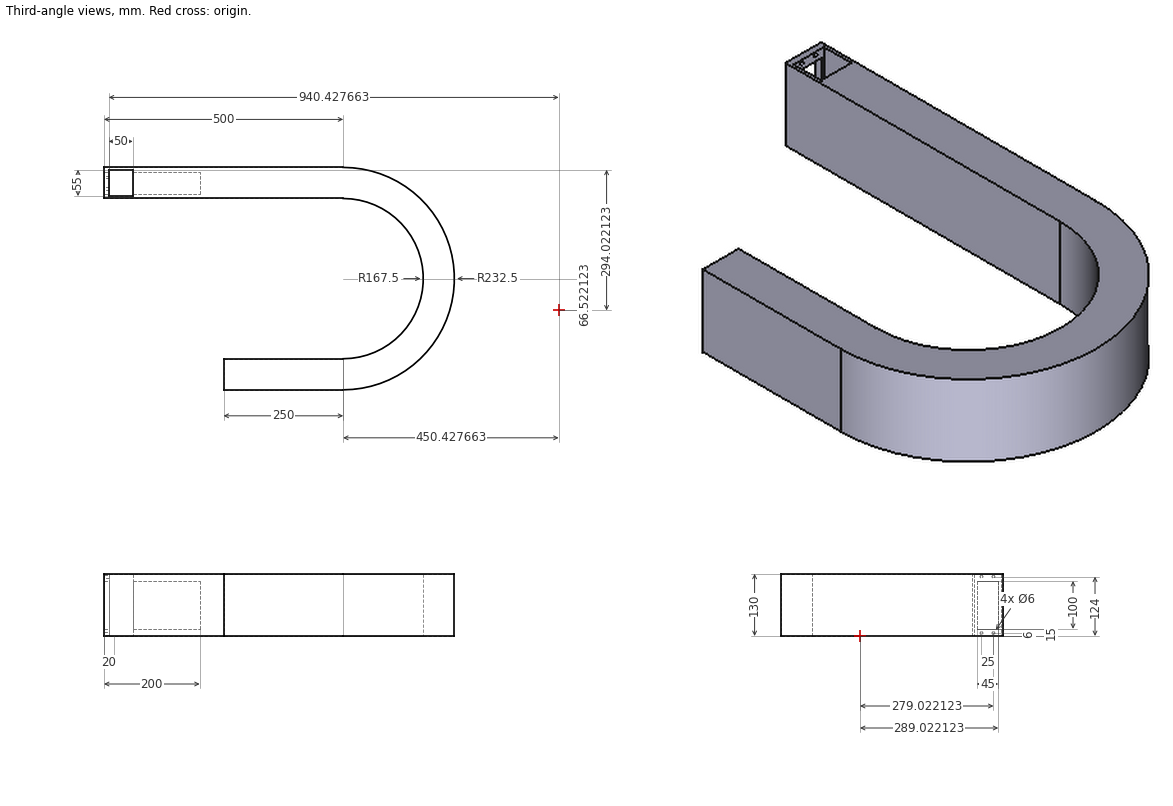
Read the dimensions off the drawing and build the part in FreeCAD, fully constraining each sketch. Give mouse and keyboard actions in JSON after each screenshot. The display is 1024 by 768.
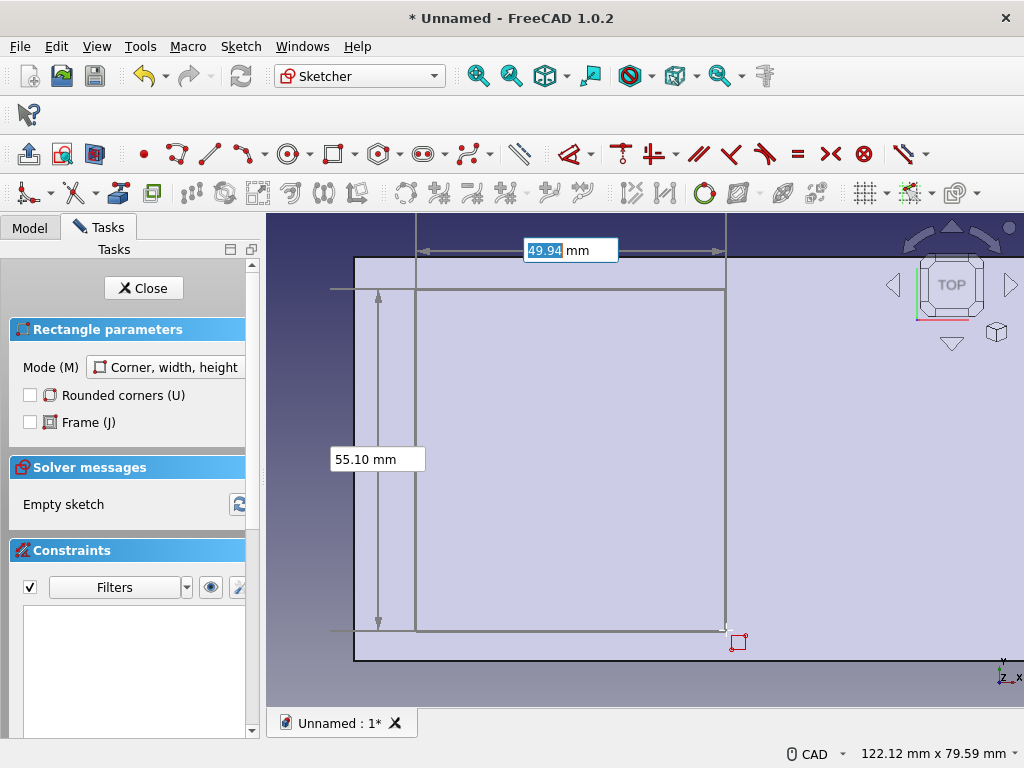
{"action": "type", "text": "50"}
{"action": "key", "text": "Tab"}
{"action": "type", "text": "55"}
{"action": "key", "text": "Return"}
{"action": "key", "text": "Escape"}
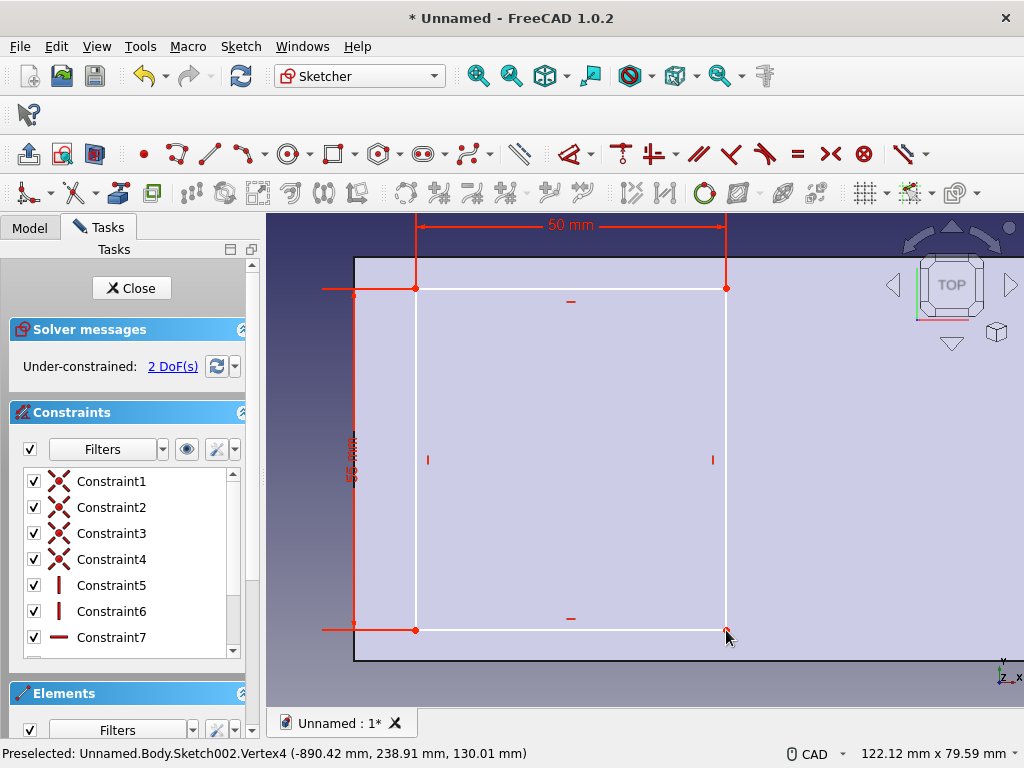
{"action": "key", "text": "d"}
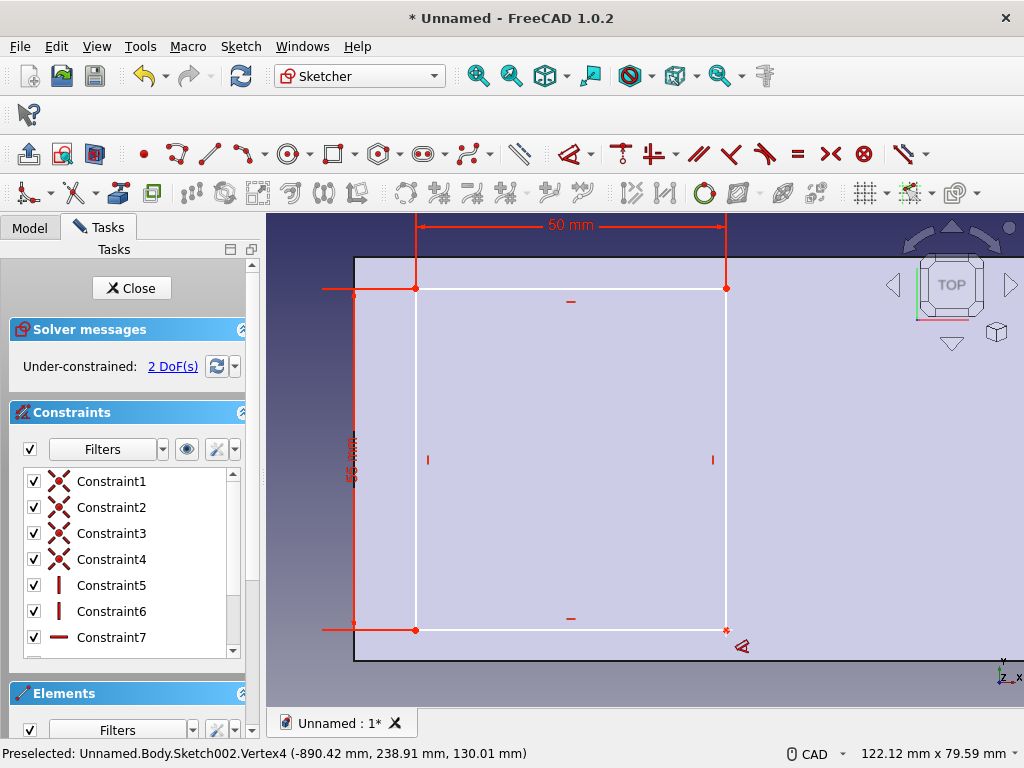
{"action": "left_click", "coordinate": [416, 289]}
{"action": "left_click", "coordinate": [637, 255]}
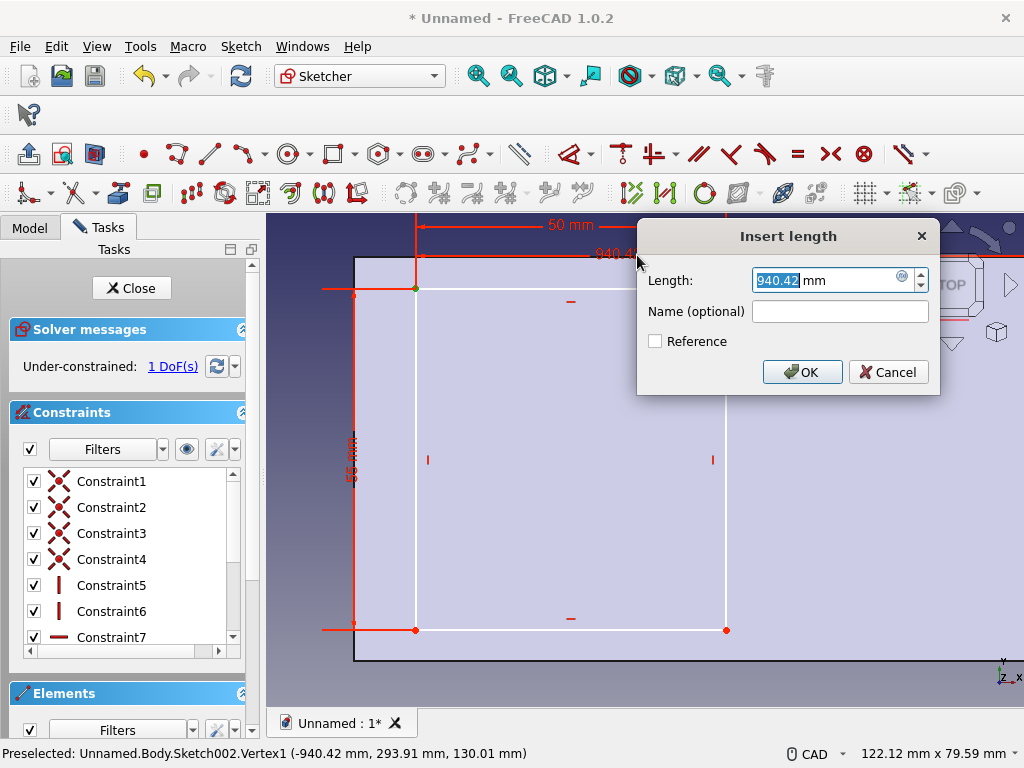
{"action": "type", "text": "940.427663"}
{"action": "key", "text": "Return"}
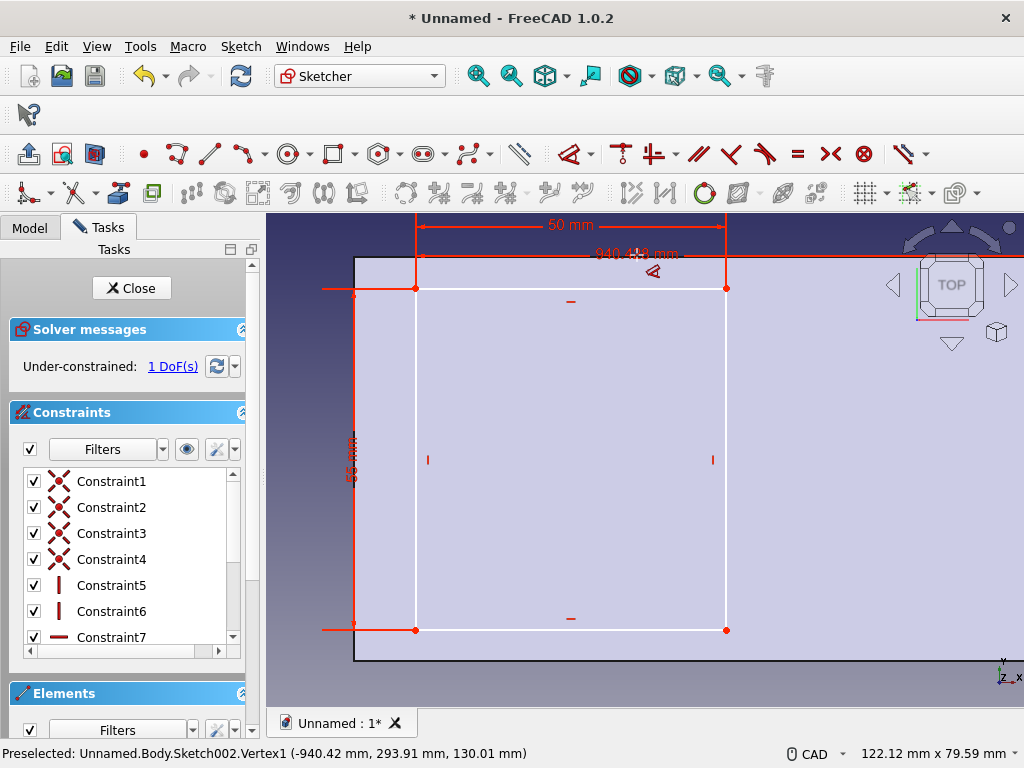
{"action": "left_click", "coordinate": [416, 289]}
{"action": "left_click", "coordinate": [382, 484]}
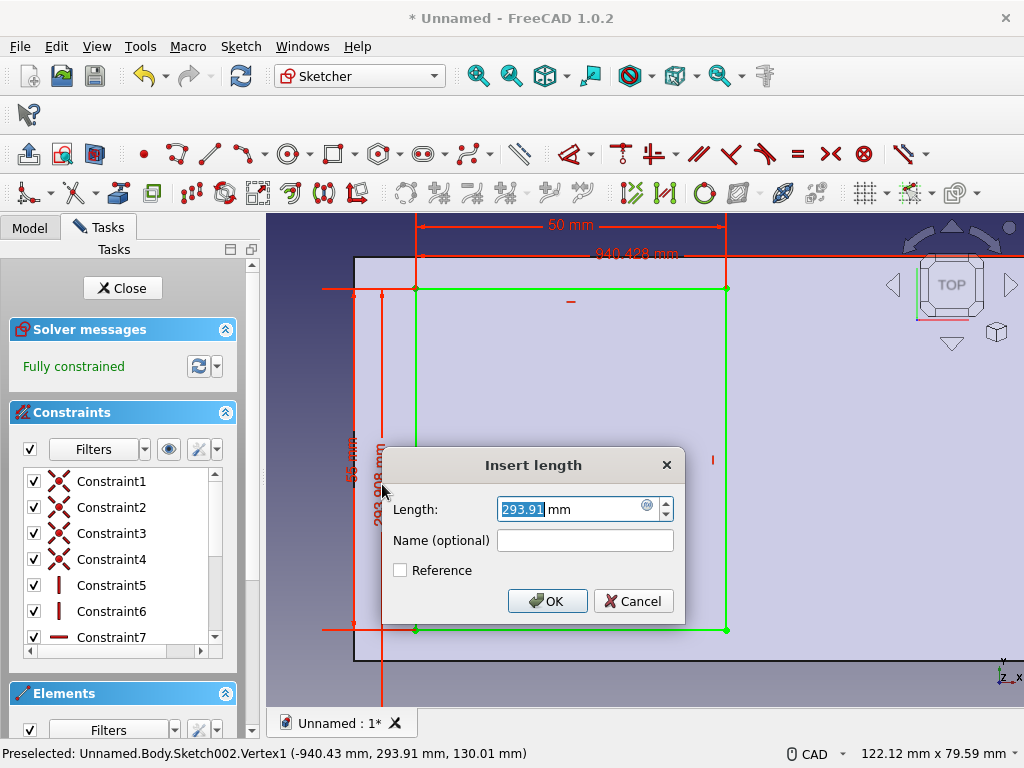
{"action": "type", "text": "294.022123"}
{"action": "key", "text": "Return"}
{"action": "key", "text": "Escape"}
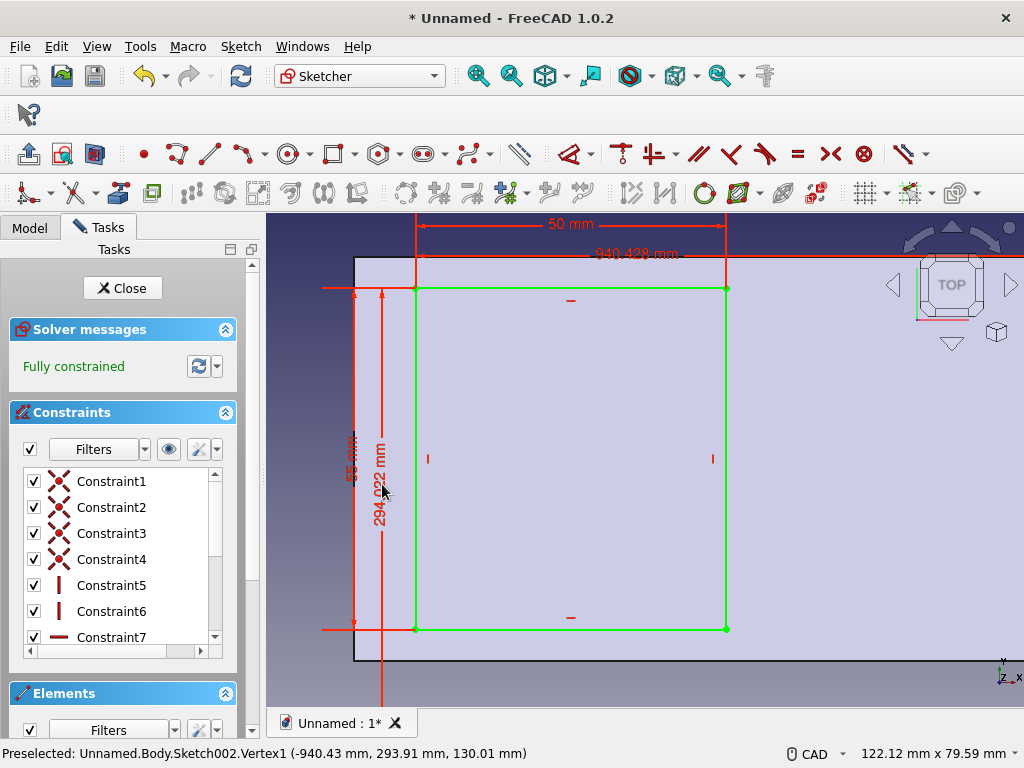
{"action": "left_click", "coordinate": [123, 288]}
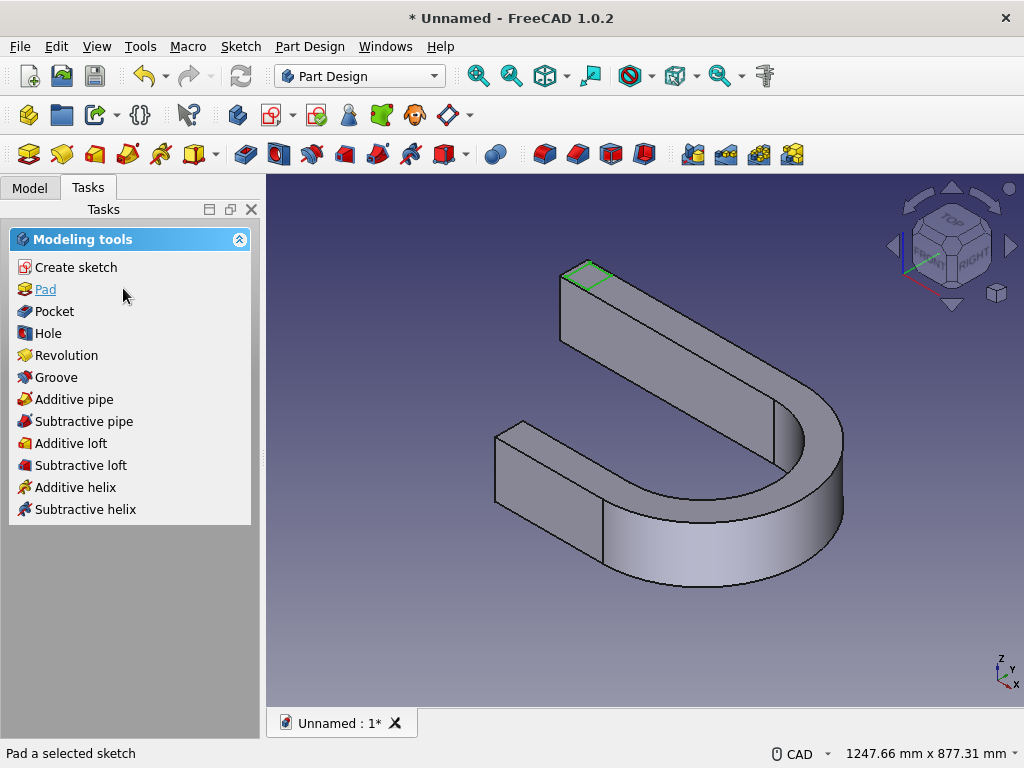
{"action": "left_click", "coordinate": [246, 154]}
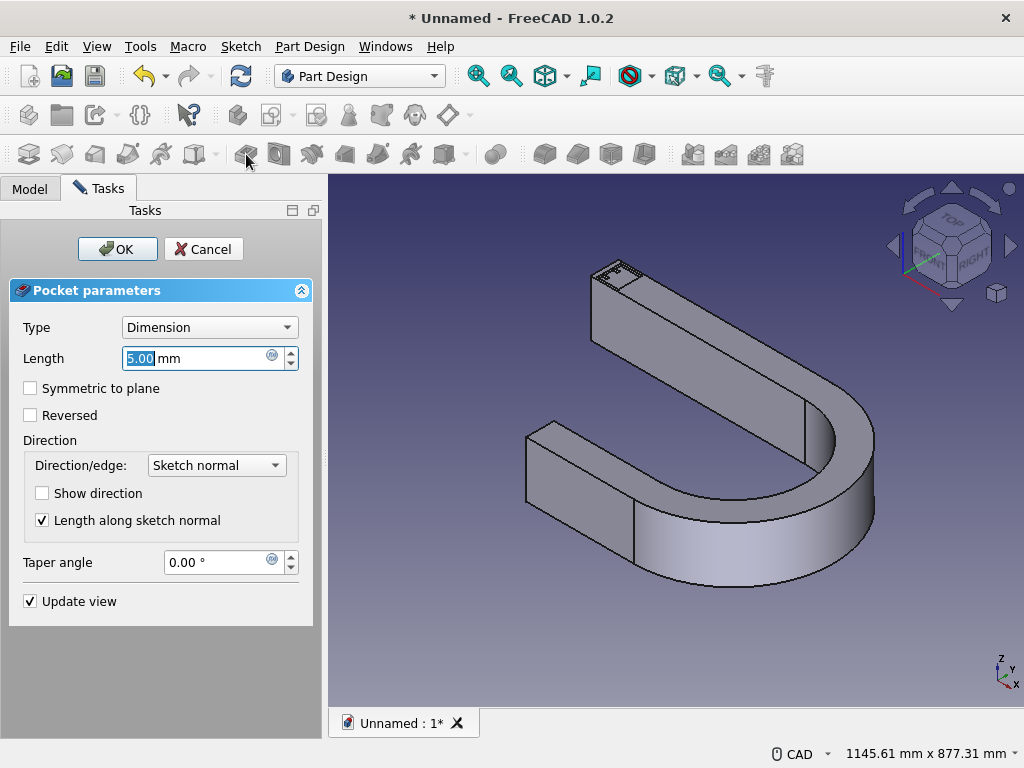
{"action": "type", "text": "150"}
{"action": "key", "text": "Tab"}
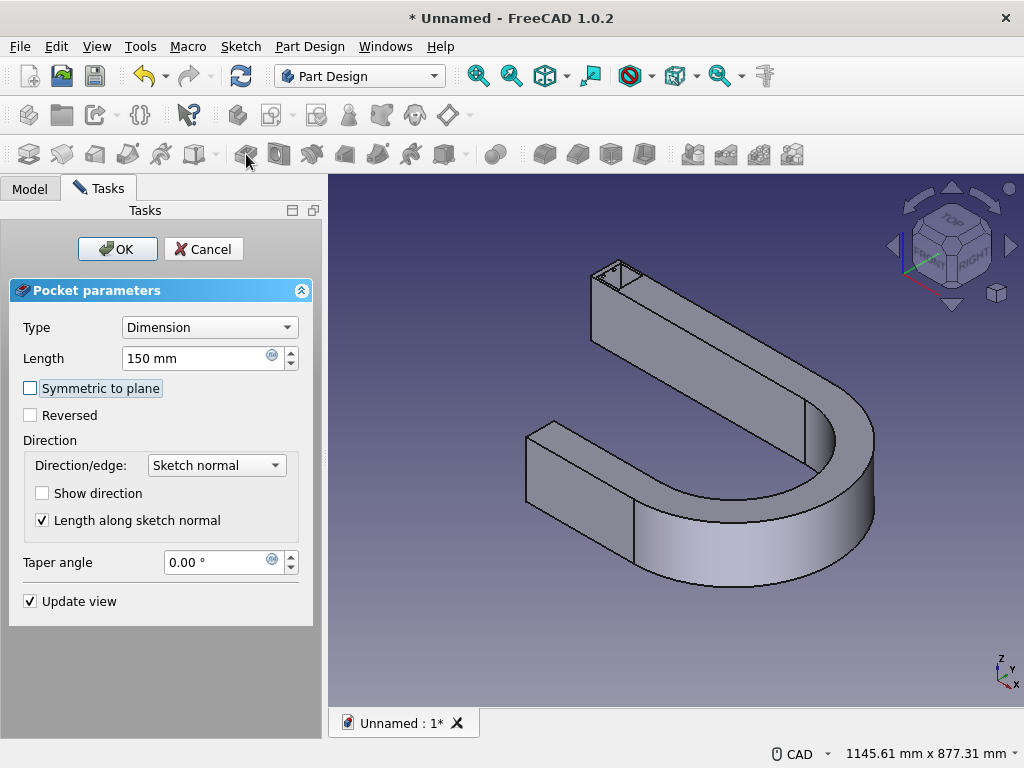
{"action": "left_click", "coordinate": [118, 249]}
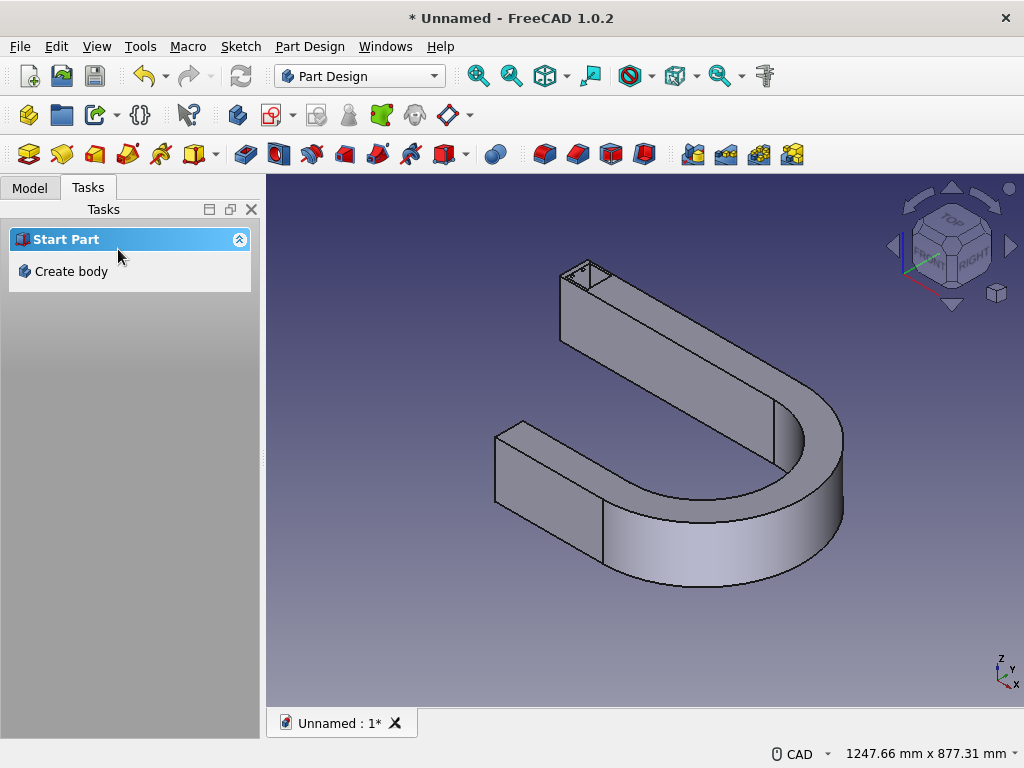
{"action": "key", "text": "6"}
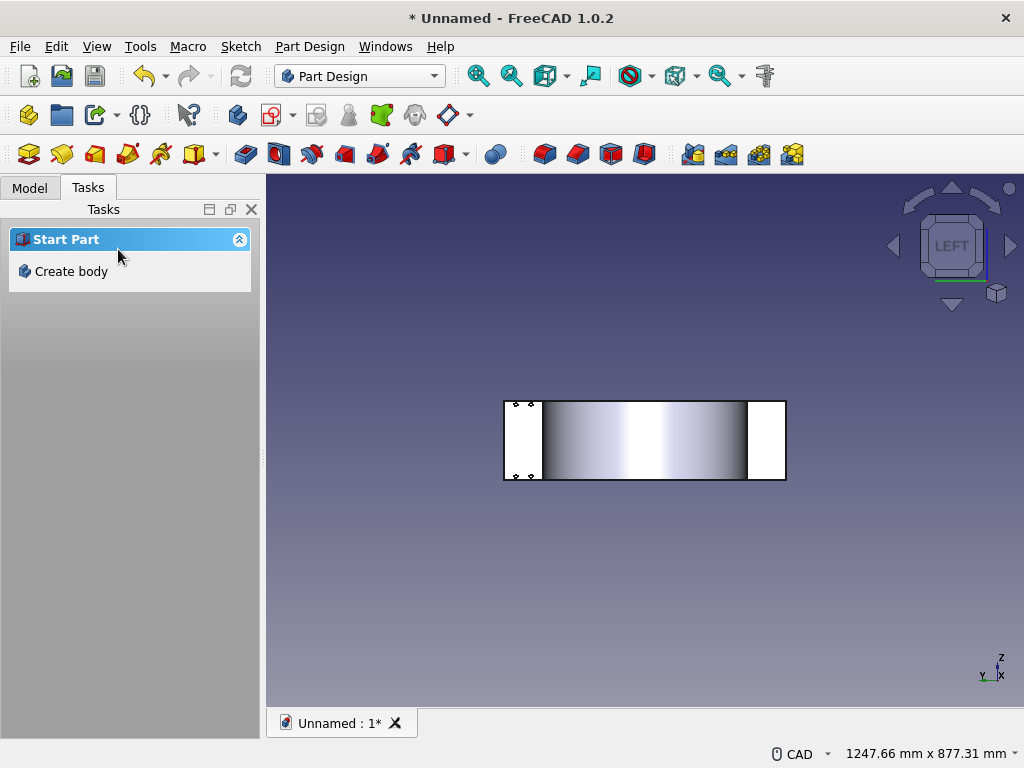
{"action": "left_click", "coordinate": [479, 76]}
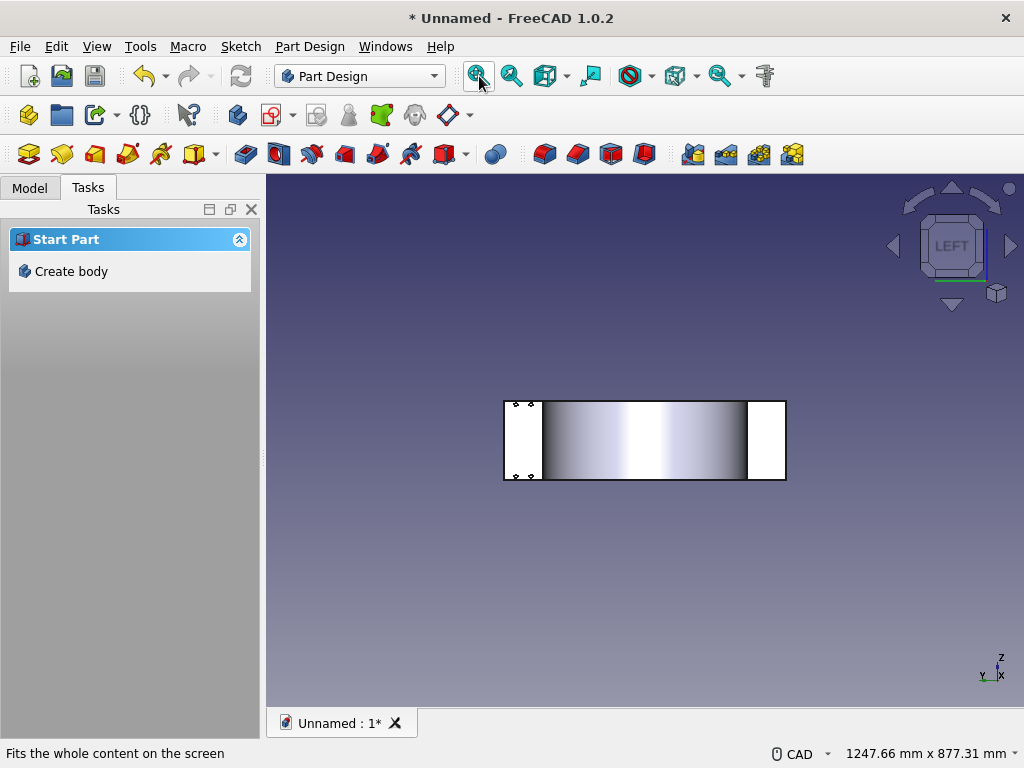
{"action": "left_click", "coordinate": [523, 428]}